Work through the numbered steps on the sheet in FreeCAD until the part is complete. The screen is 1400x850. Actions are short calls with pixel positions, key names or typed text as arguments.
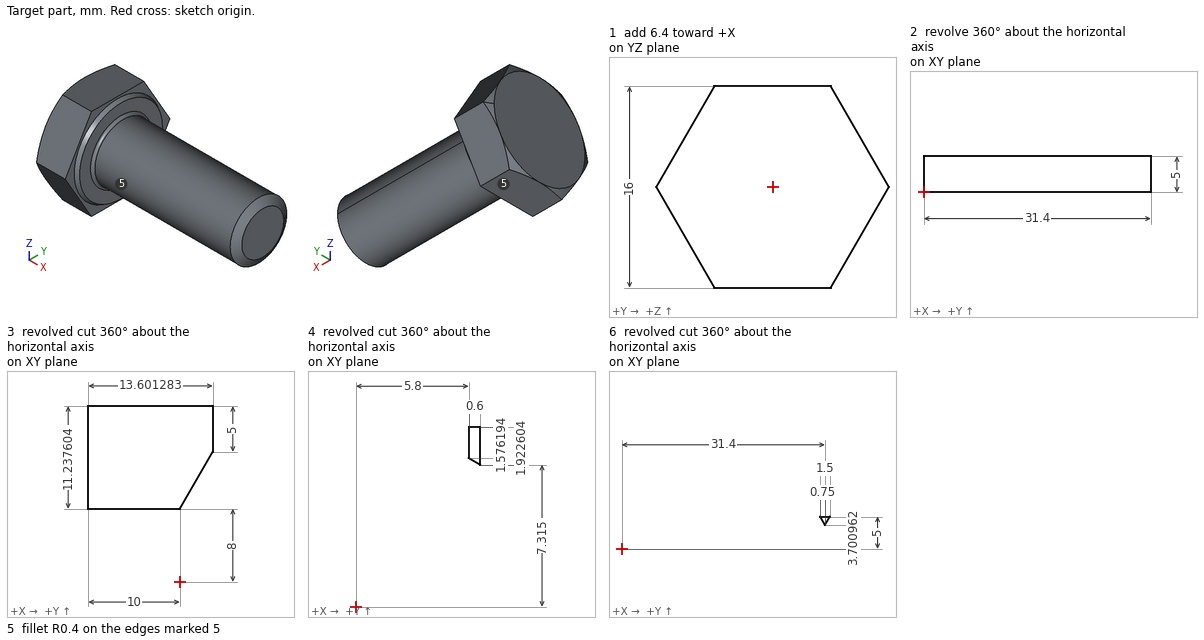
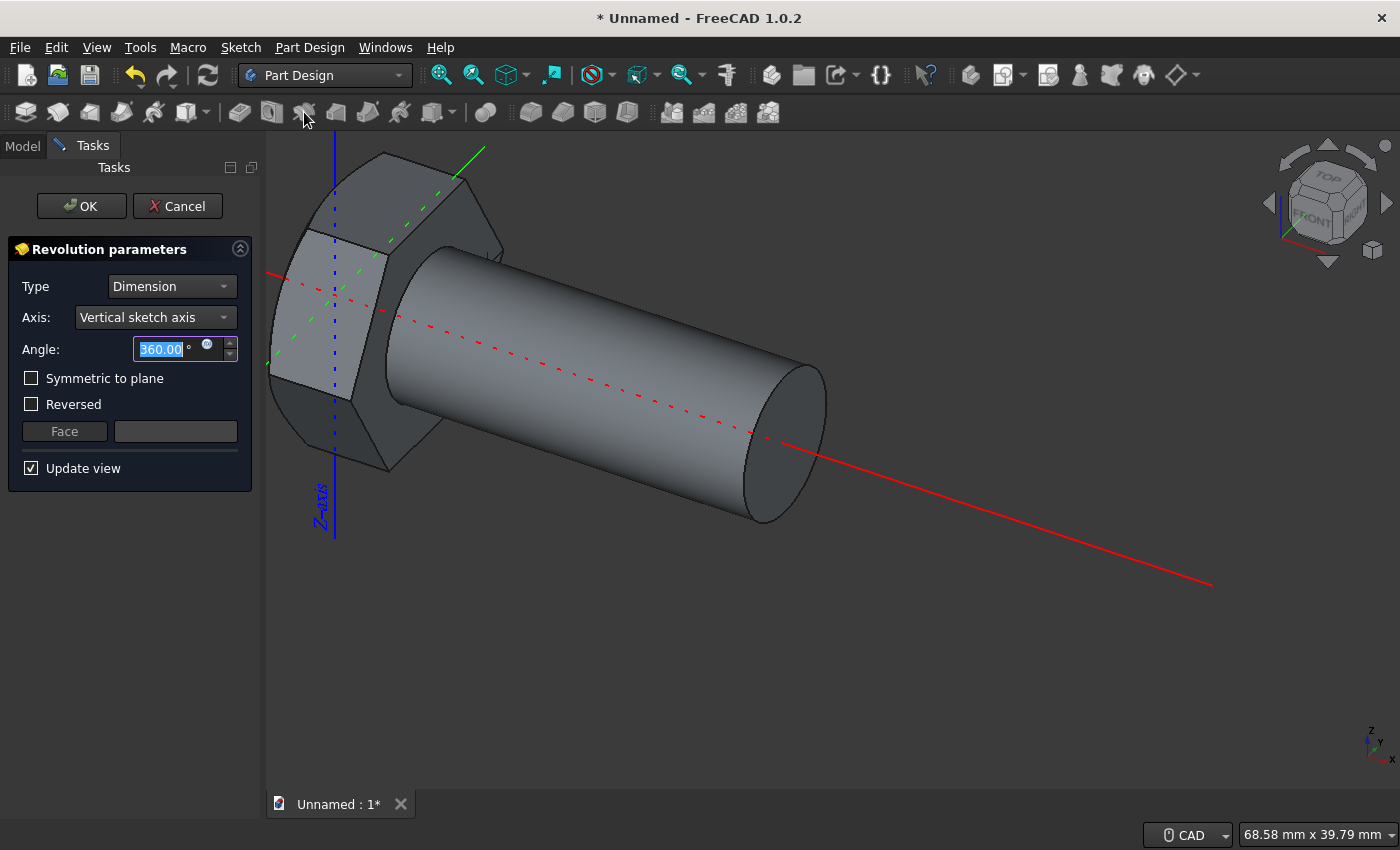
click(156, 318)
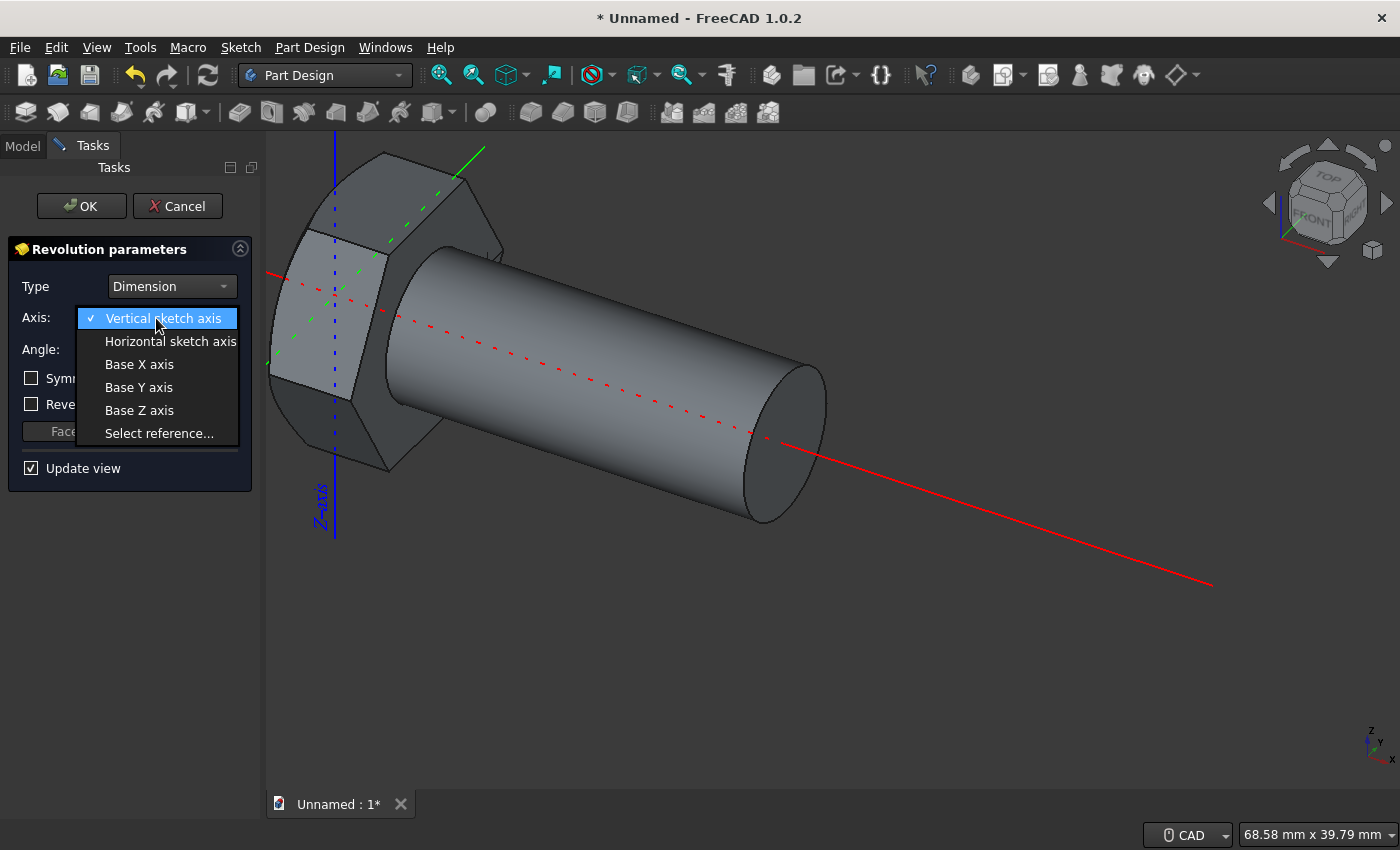
click(156, 342)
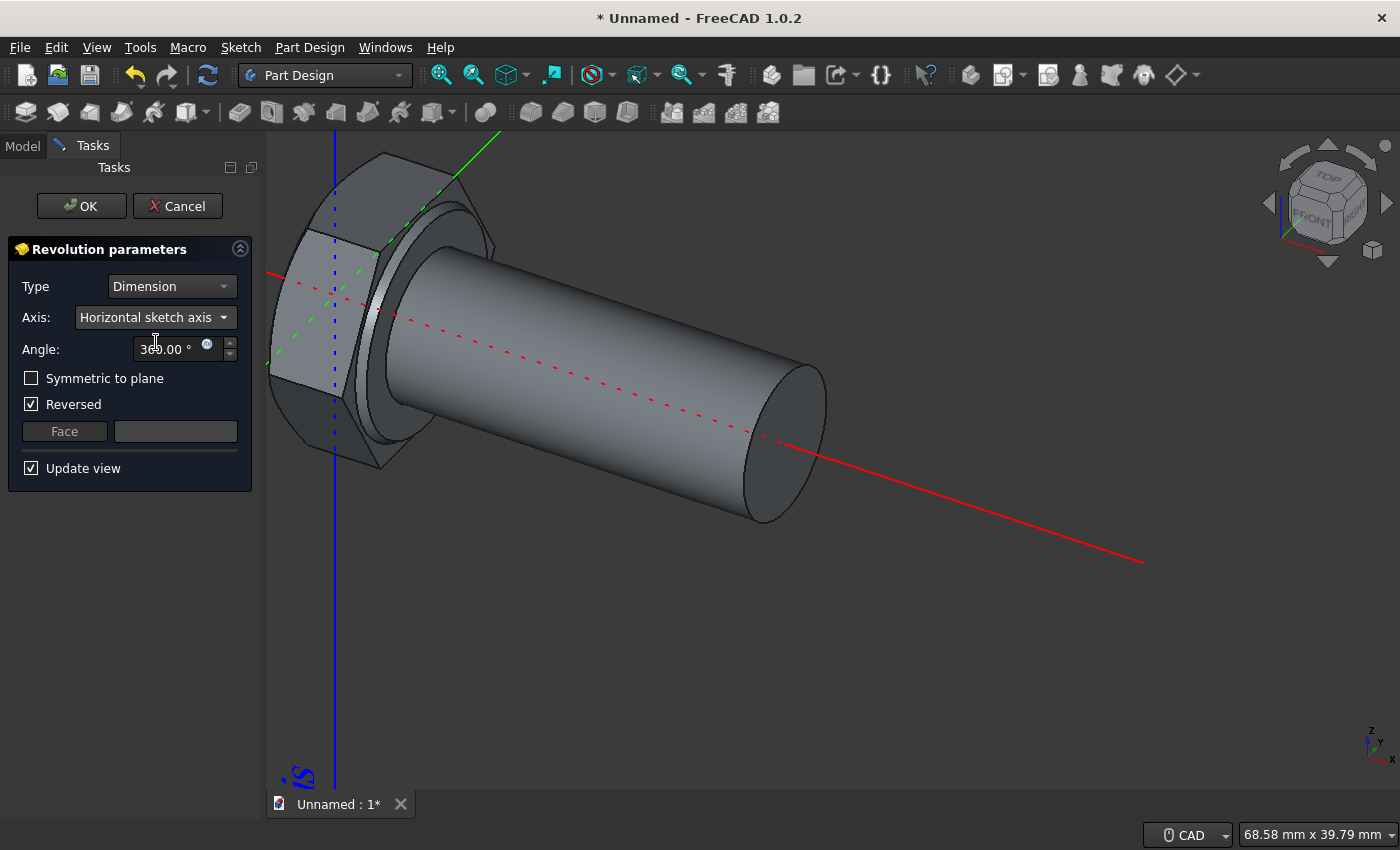
click(82, 206)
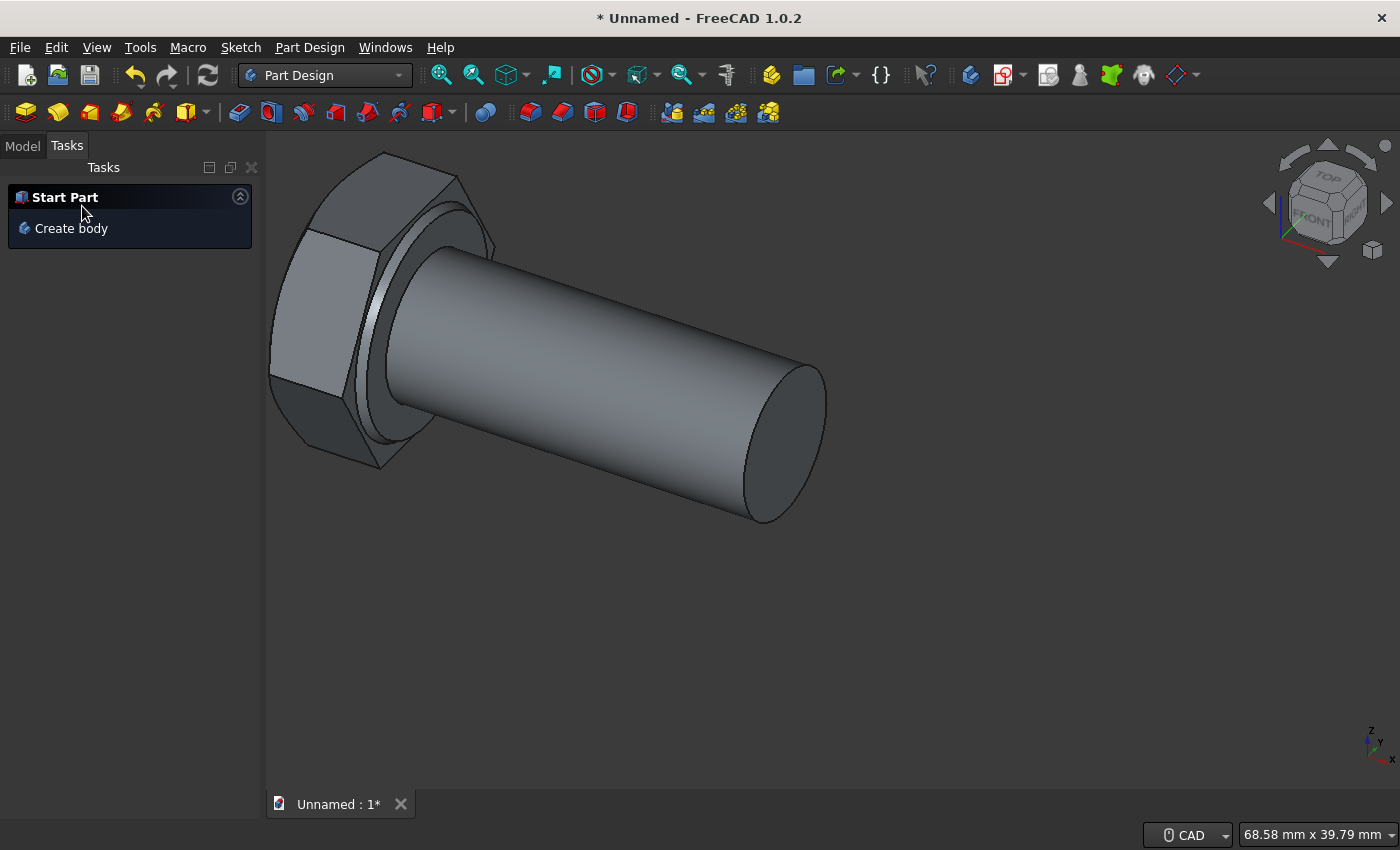
click(442, 76)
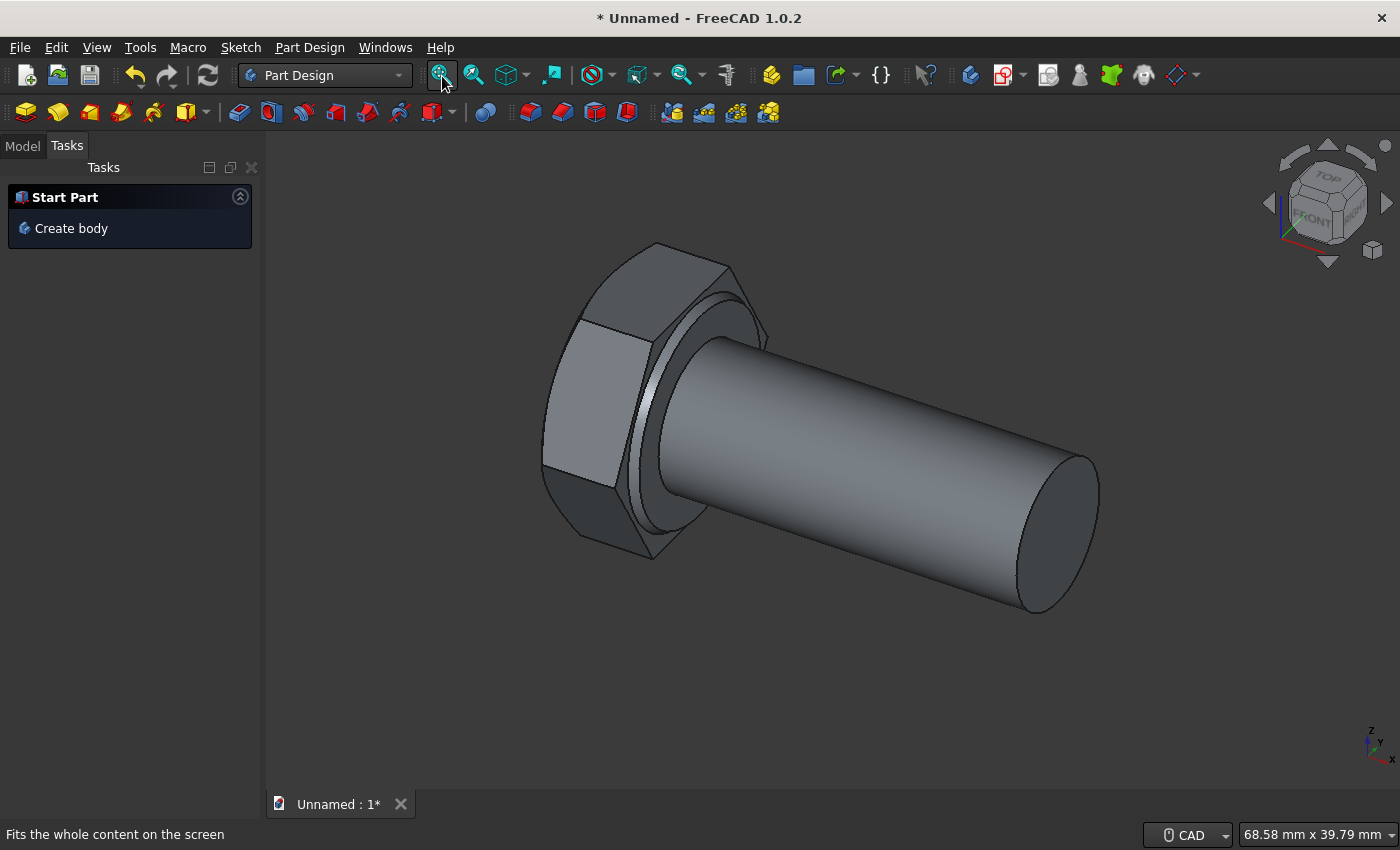
key(0)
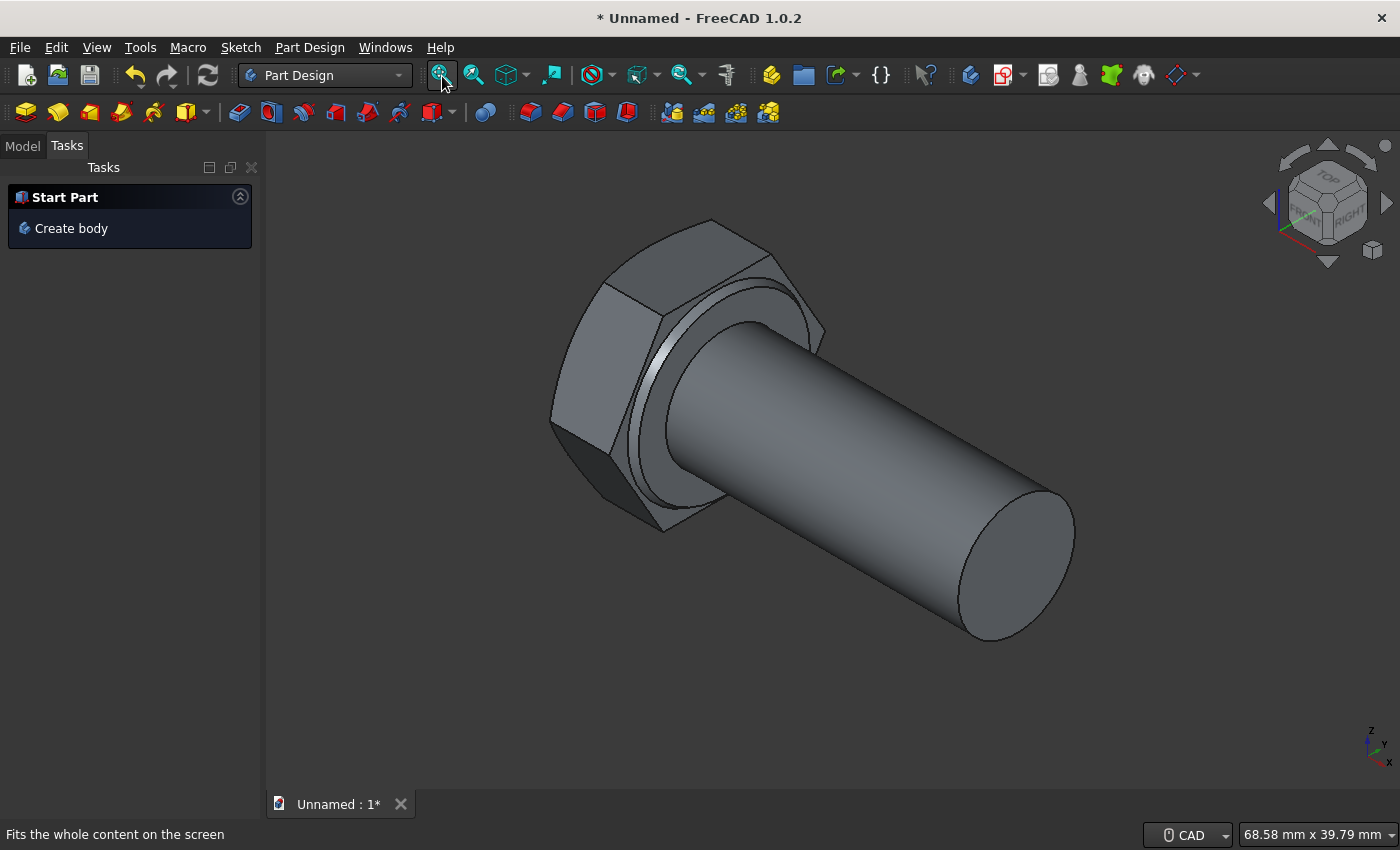
key(2)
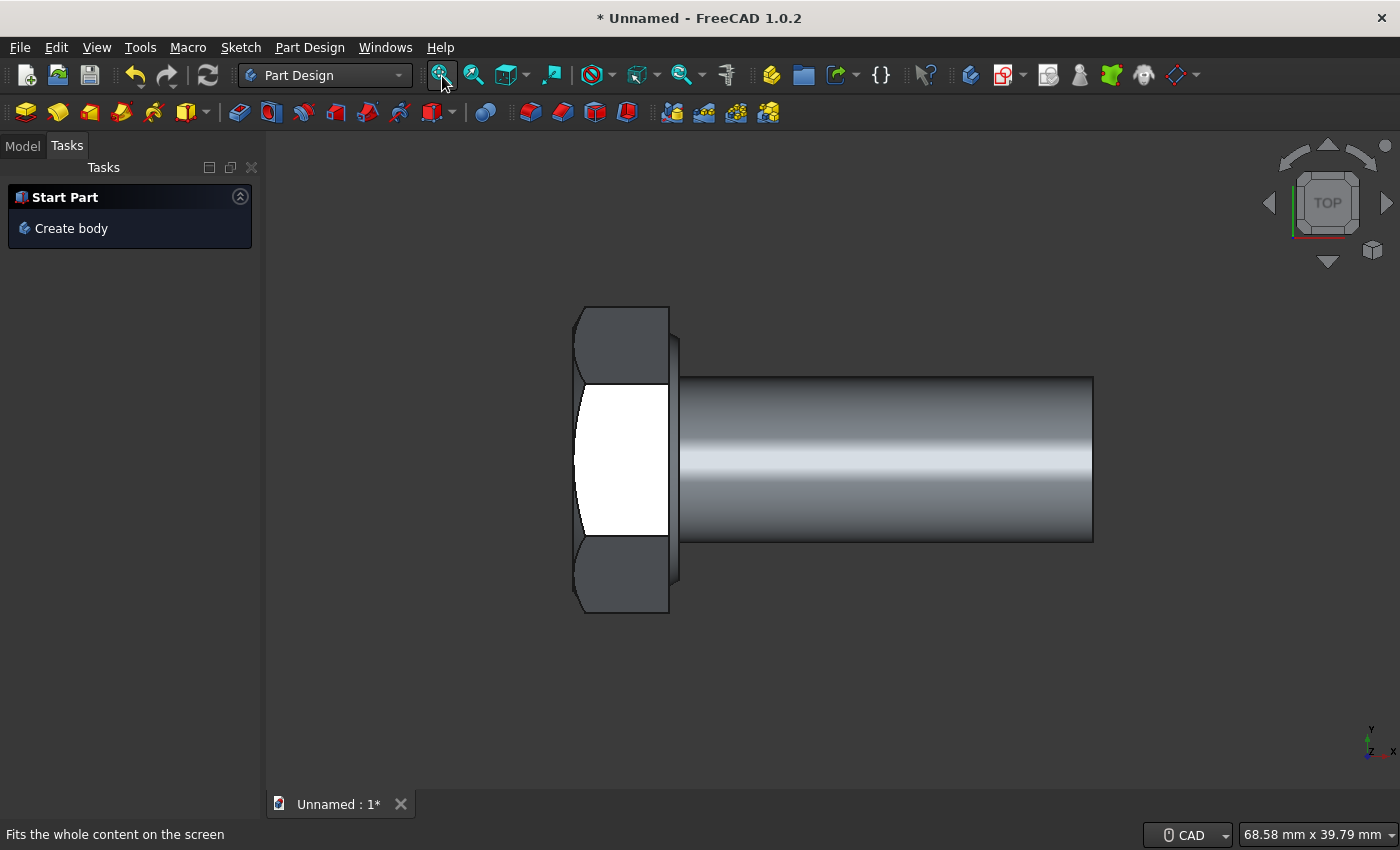
key(1)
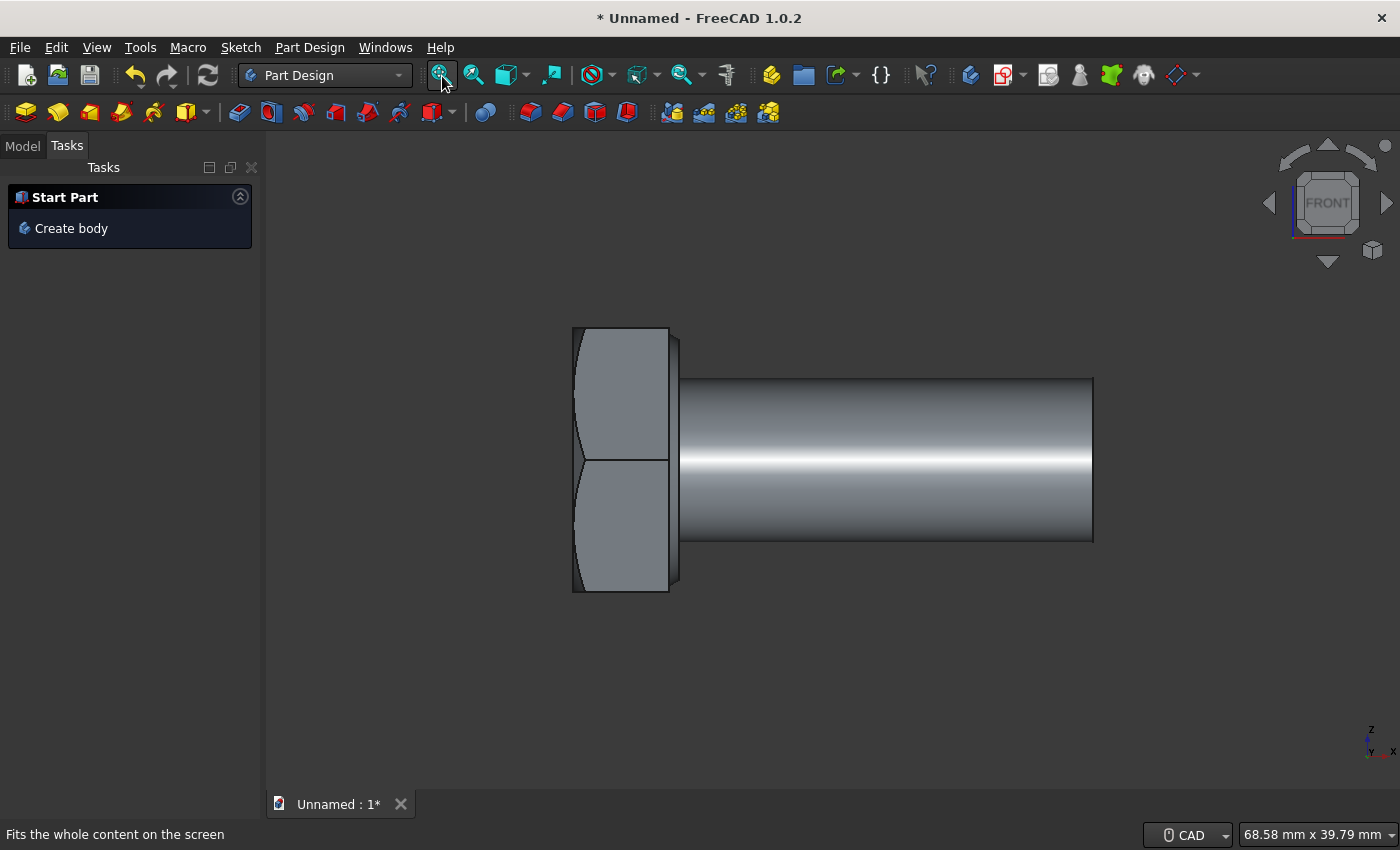
key(3)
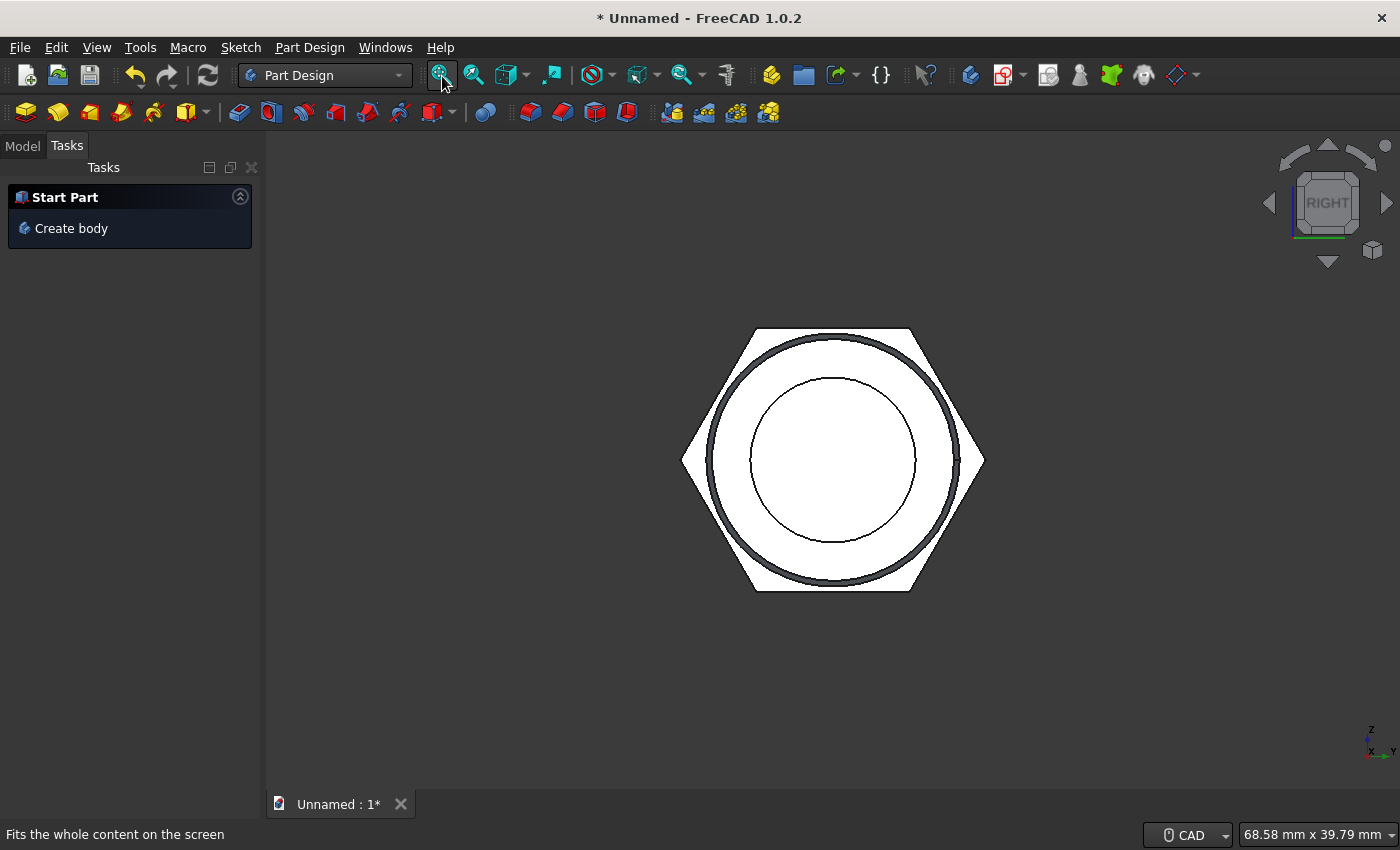
click(442, 76)